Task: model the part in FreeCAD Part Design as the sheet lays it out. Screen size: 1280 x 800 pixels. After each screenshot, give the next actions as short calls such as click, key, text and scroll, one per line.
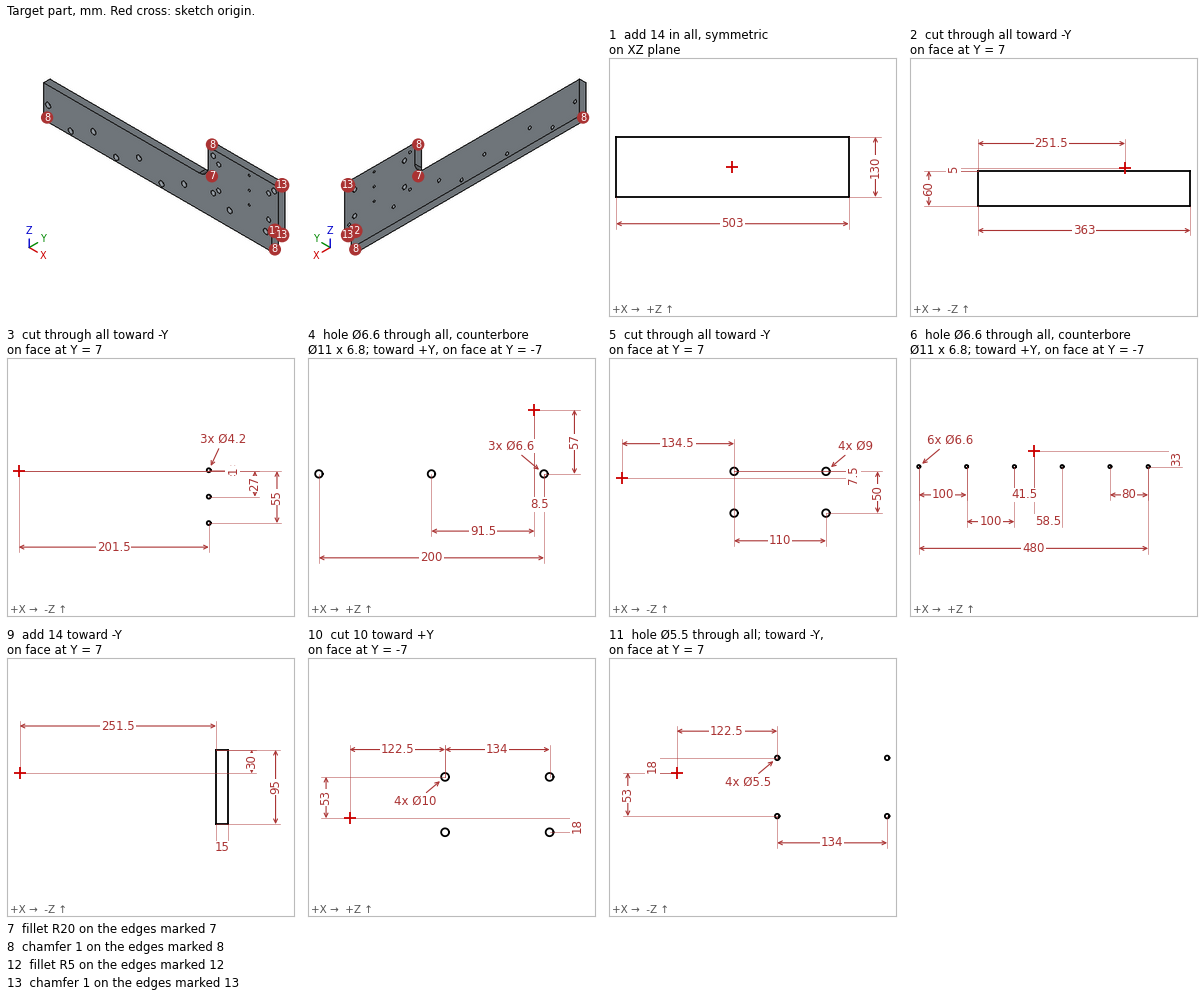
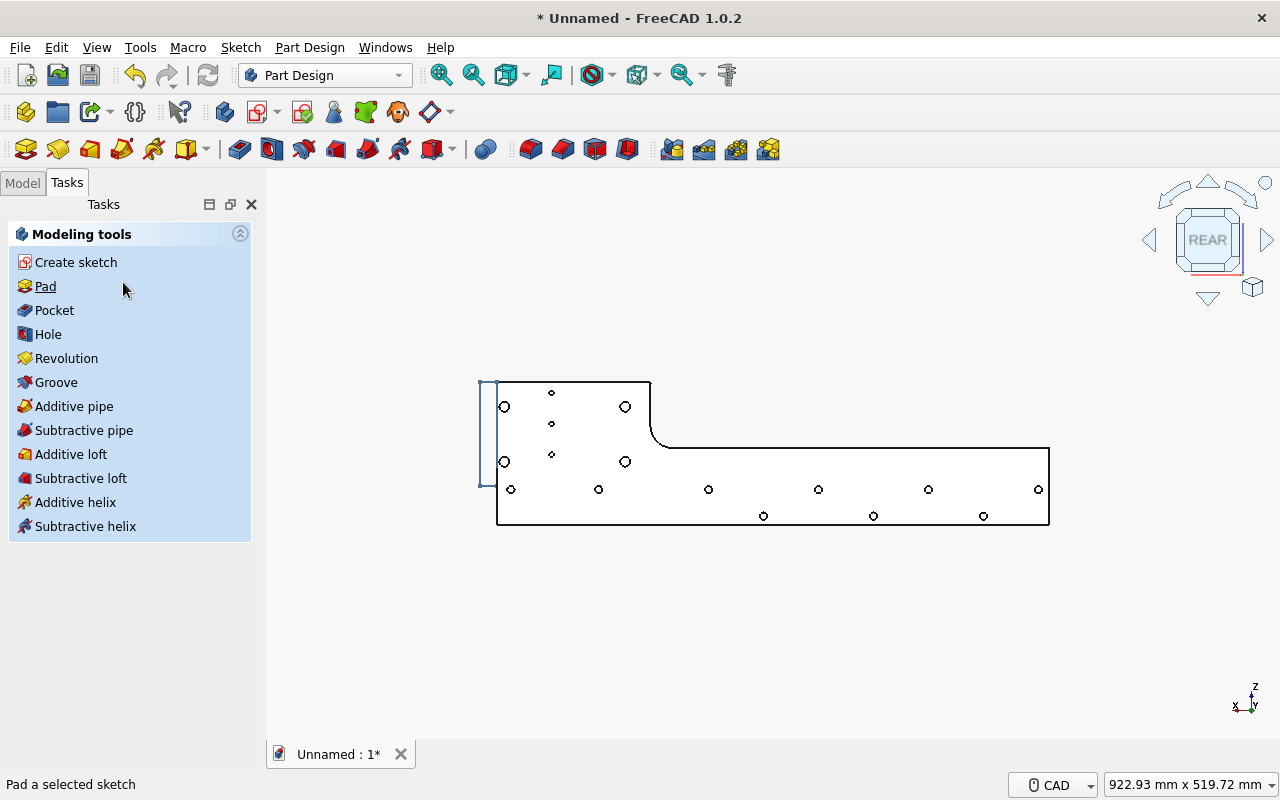
click(26, 150)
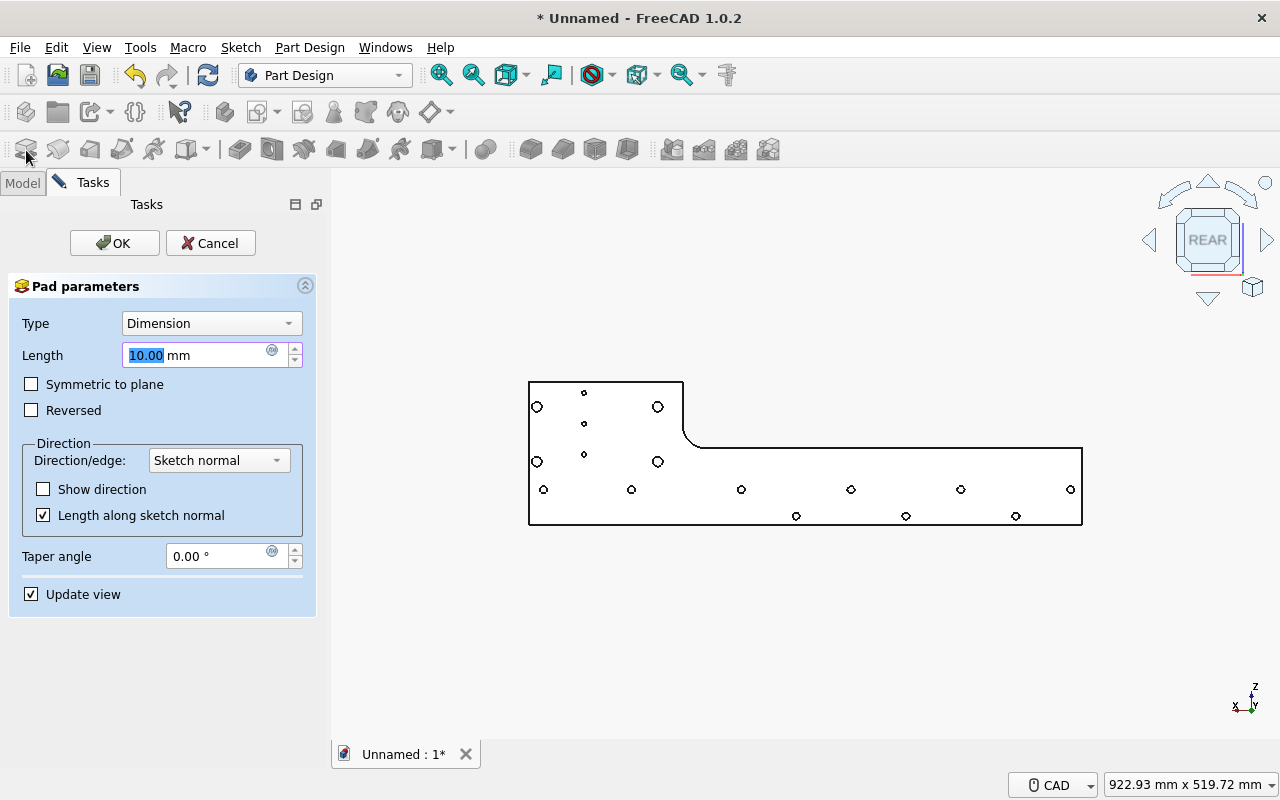
text(14)
key(Tab)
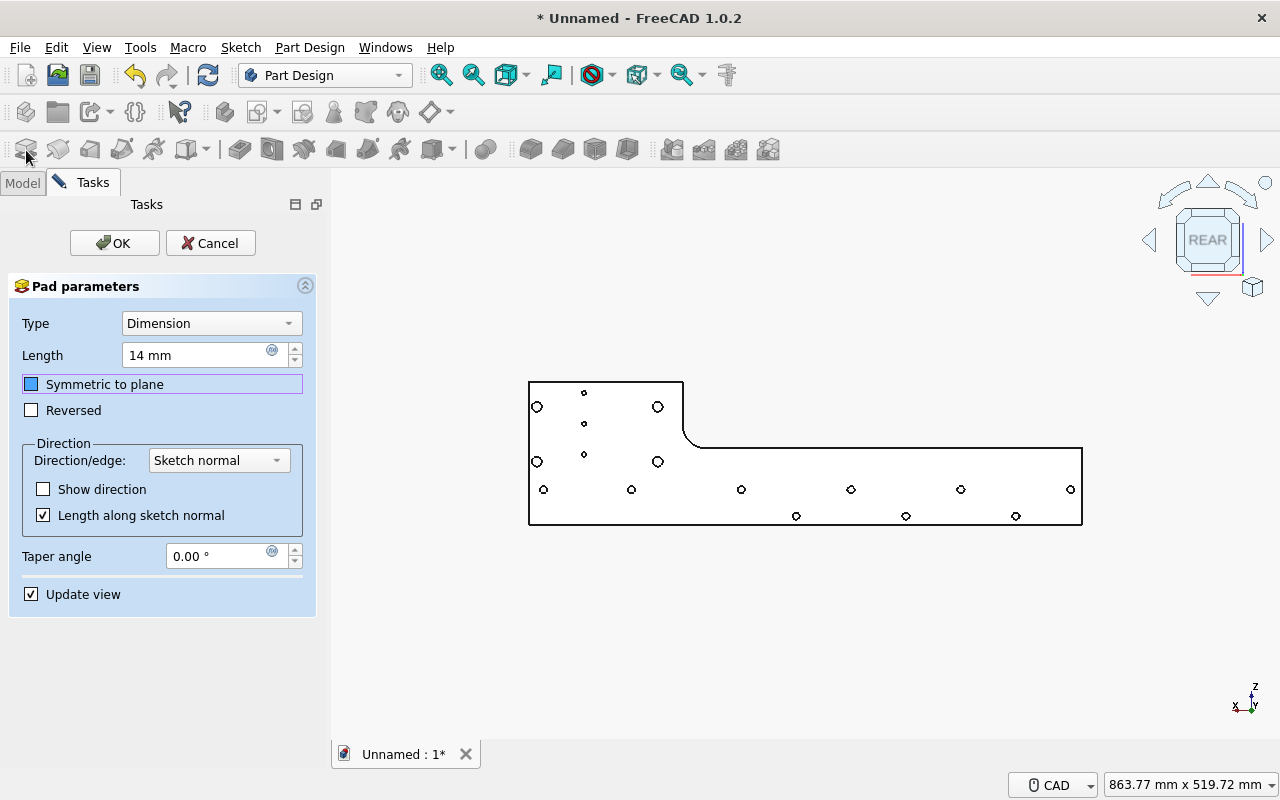
click(30, 410)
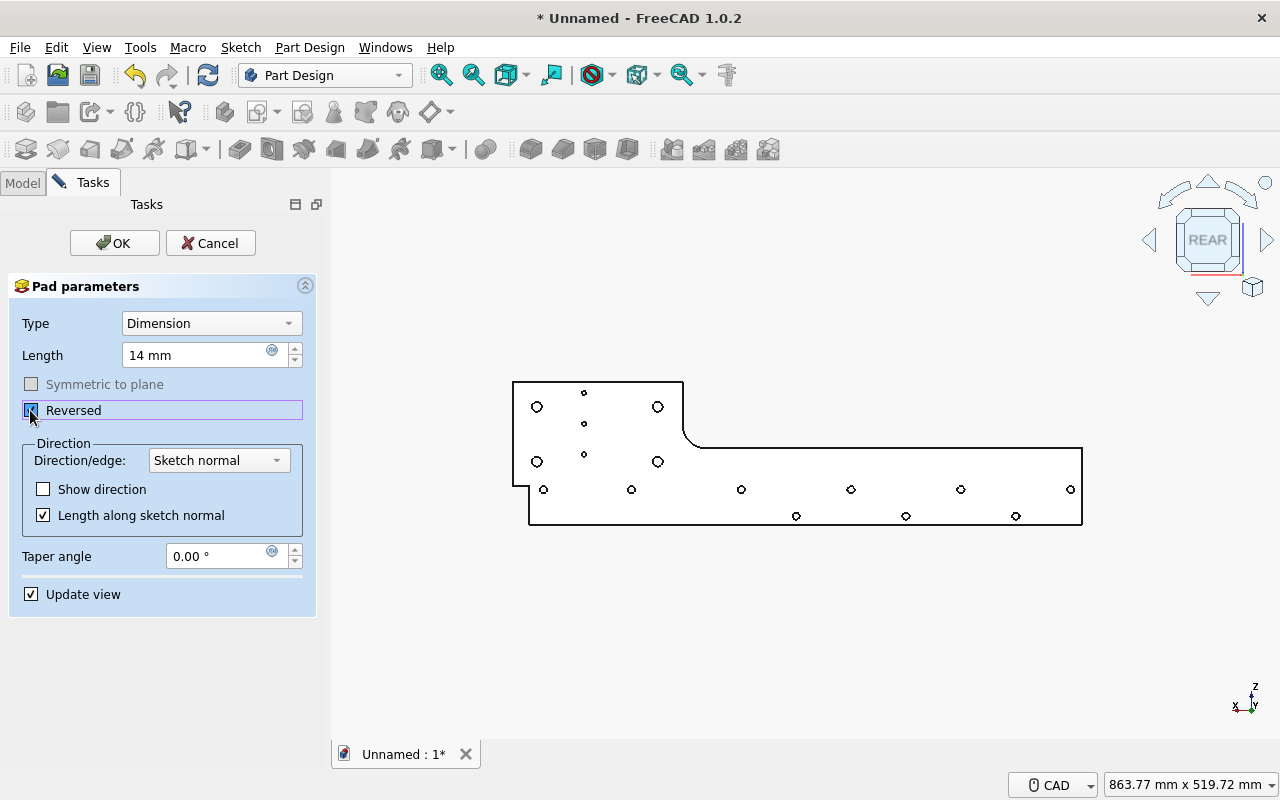
click(115, 243)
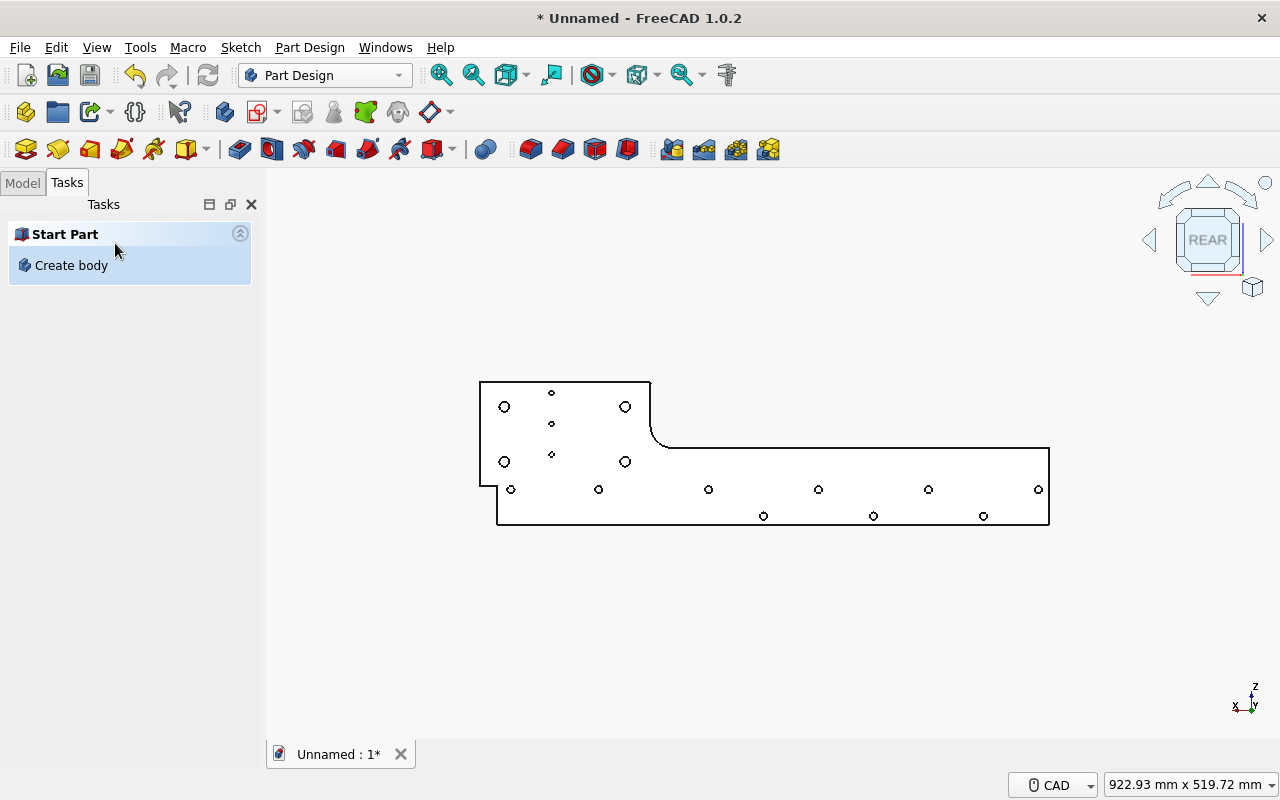
key(0)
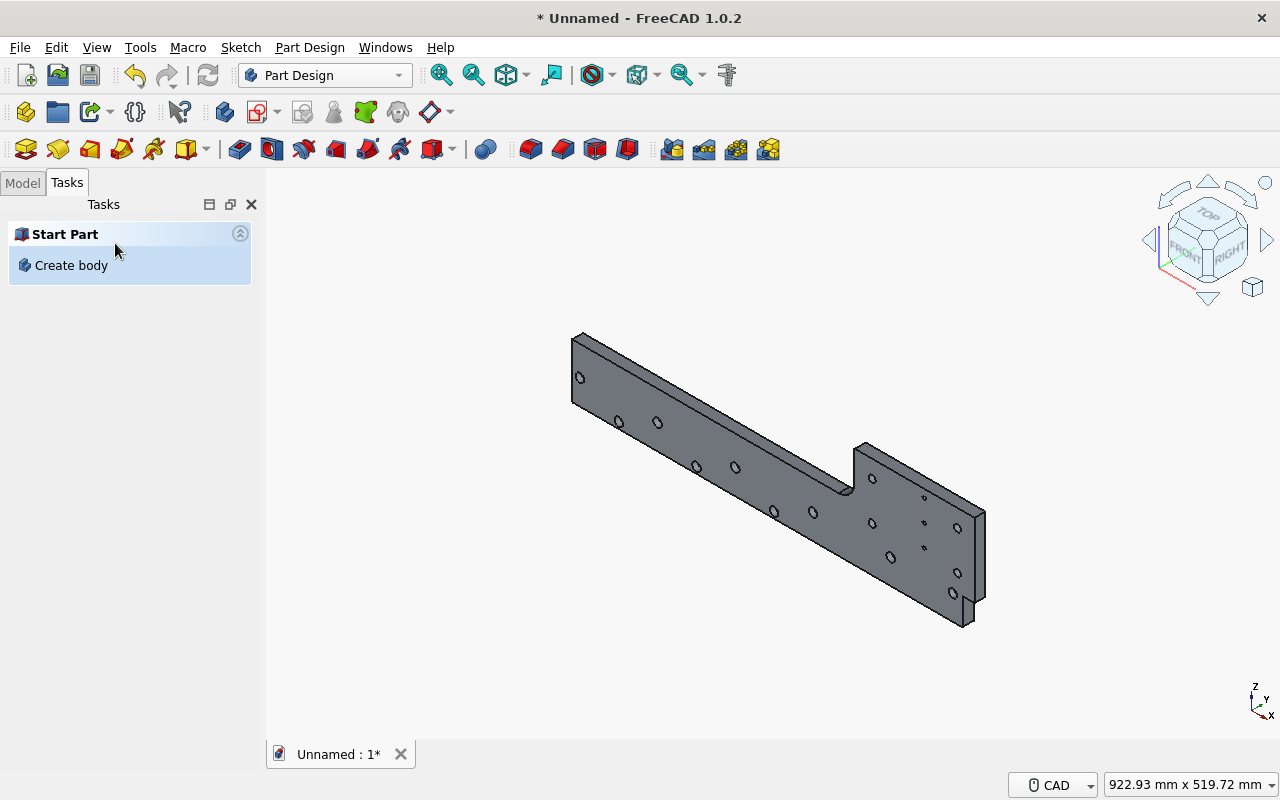
click(888, 509)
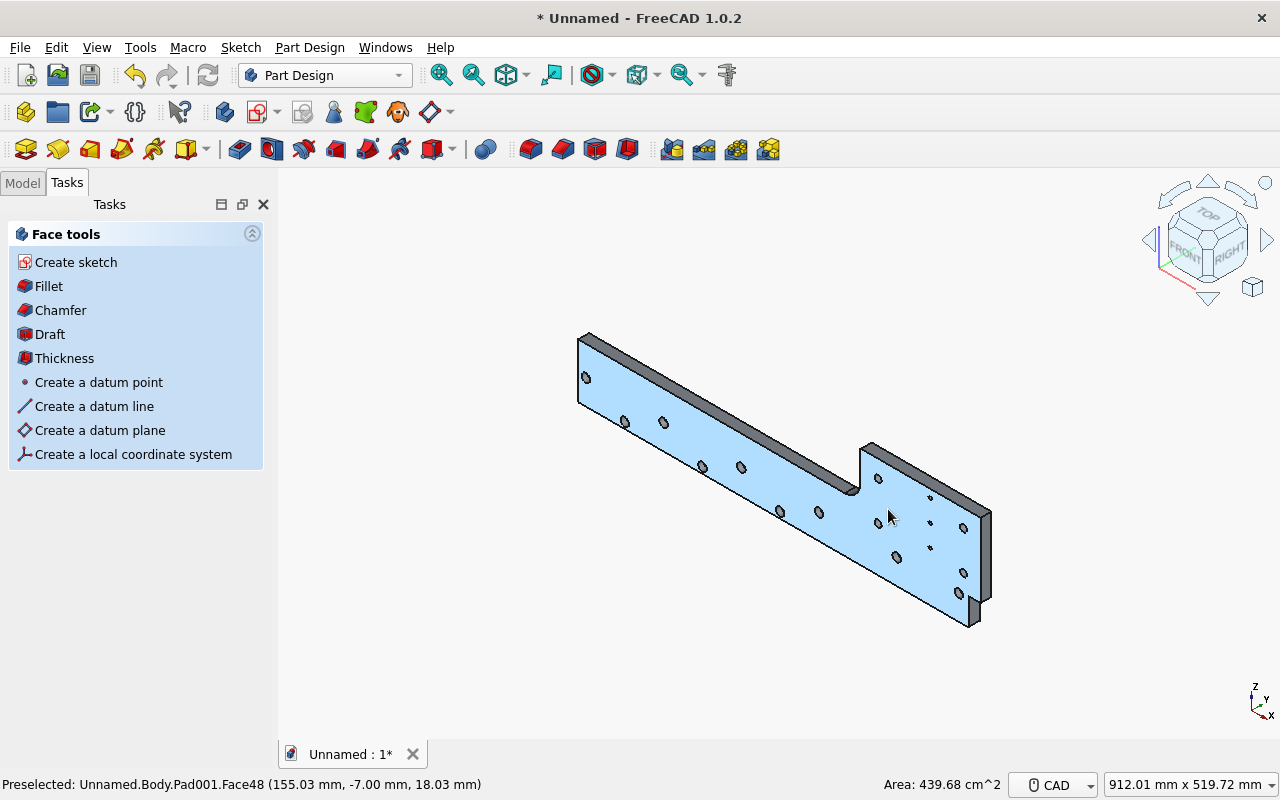
click(258, 112)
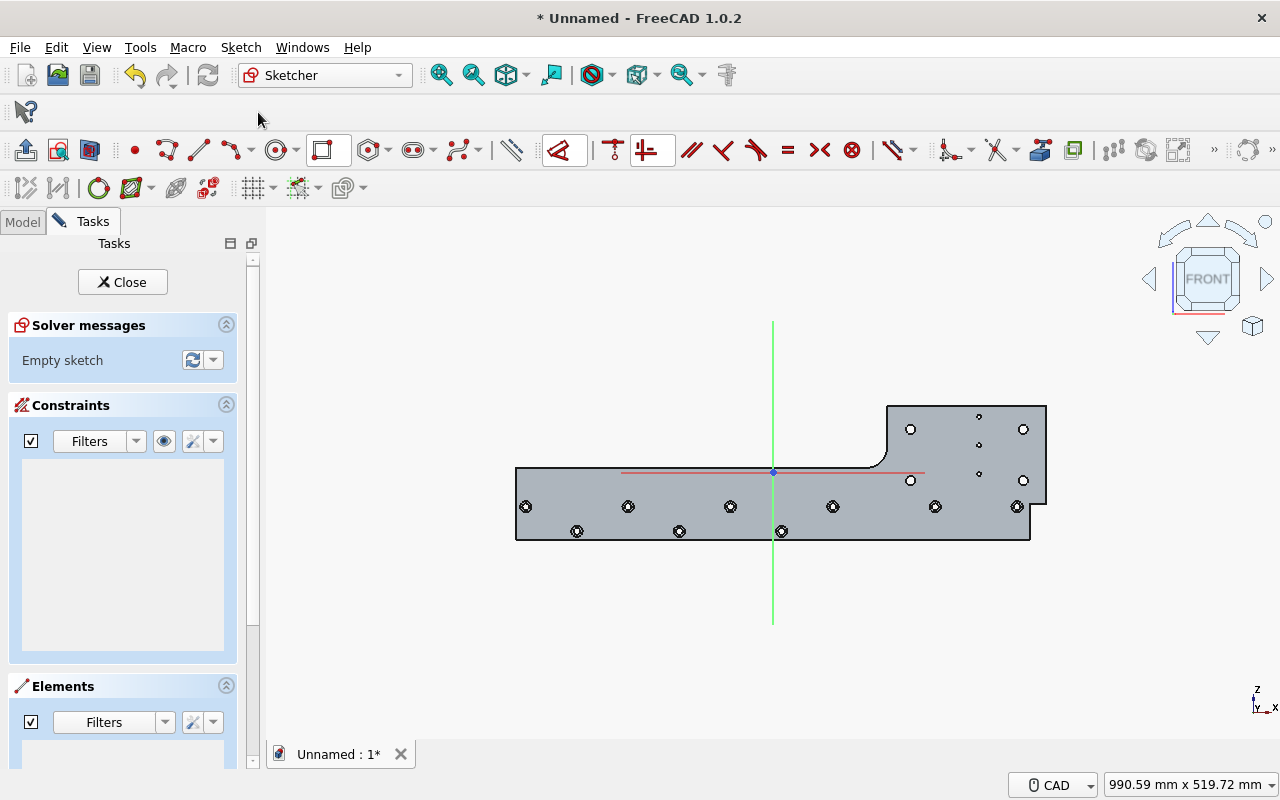
scroll(1072, 440, up, 4)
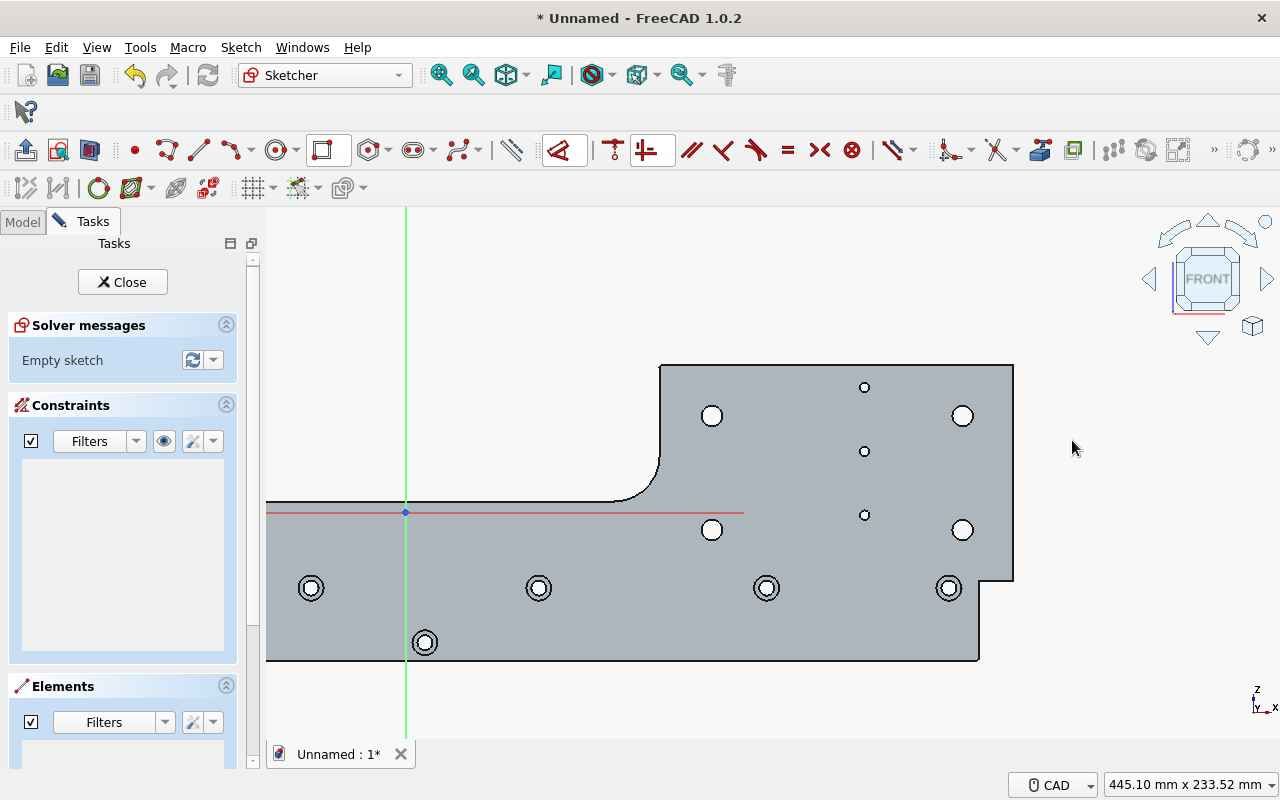
key(g)
key(c)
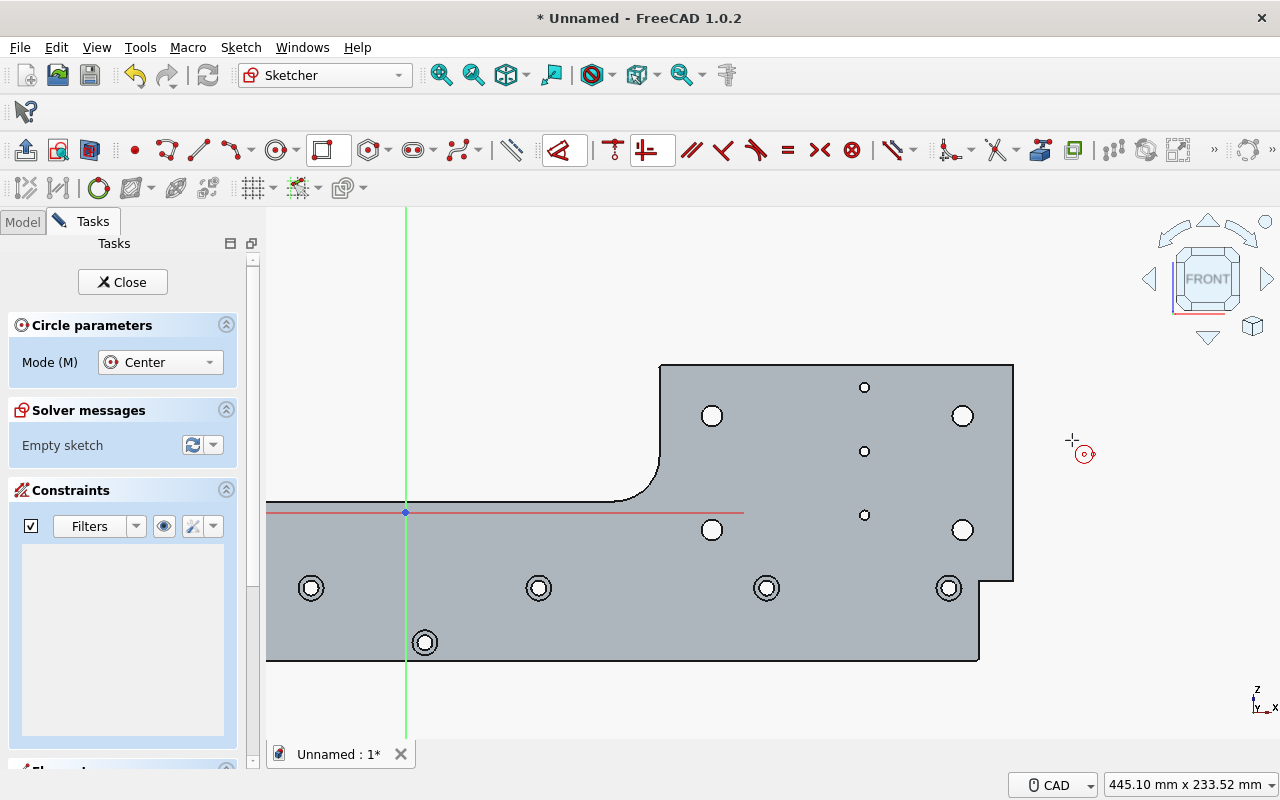
scroll(685, 392, up, 4)